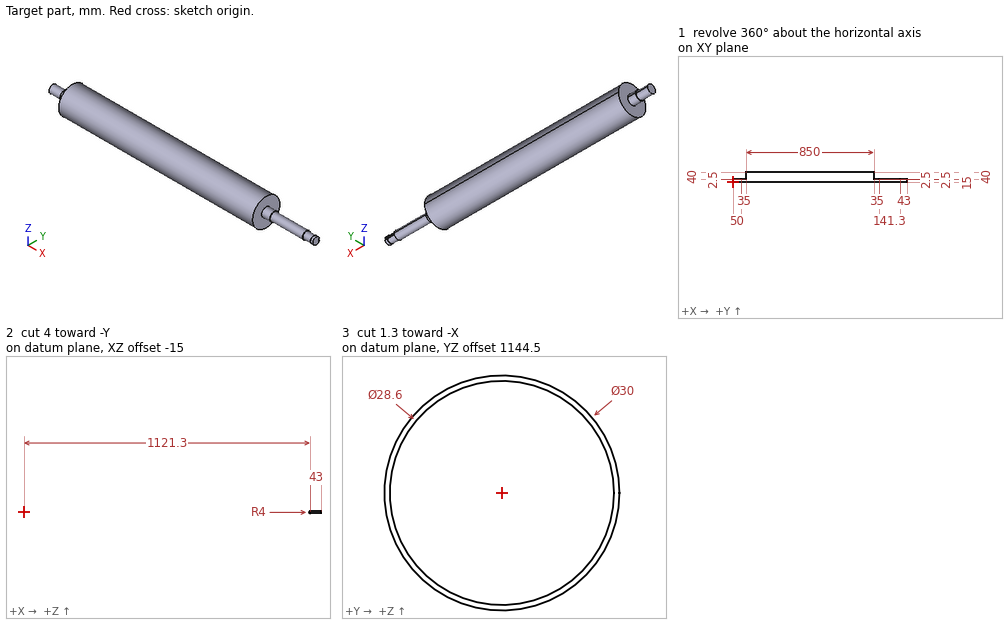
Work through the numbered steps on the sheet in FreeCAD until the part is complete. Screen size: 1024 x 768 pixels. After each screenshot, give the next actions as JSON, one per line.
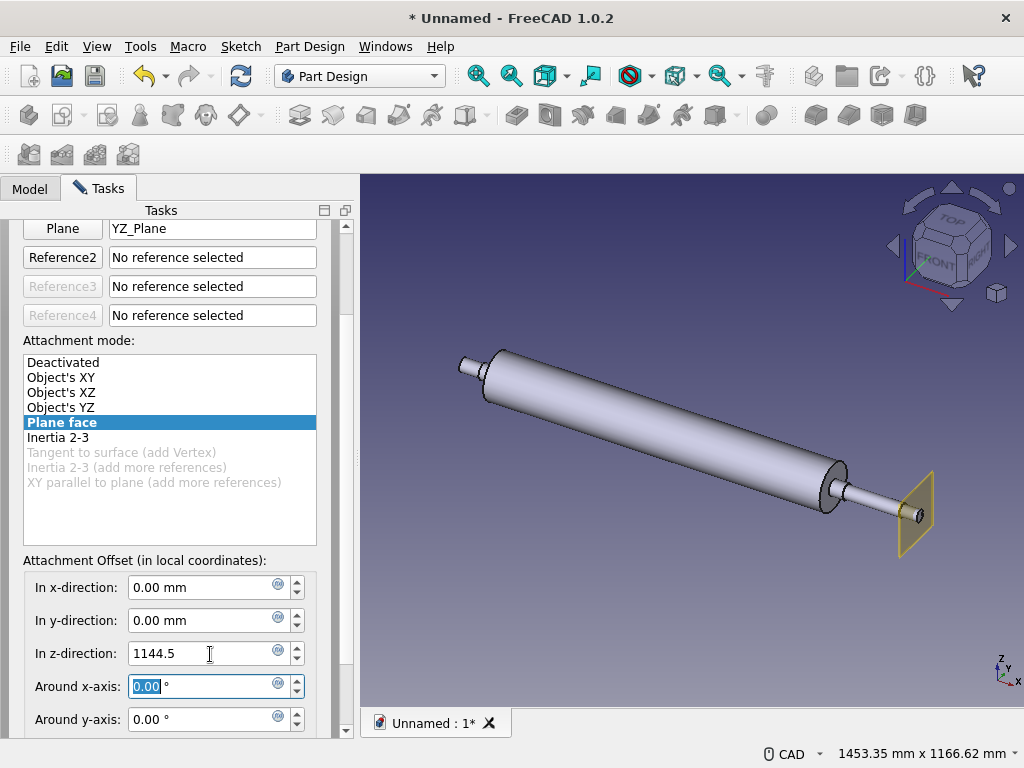
{"action": "scroll", "coordinate": [346, 479], "scroll_direction": "up", "scroll_amount": 3}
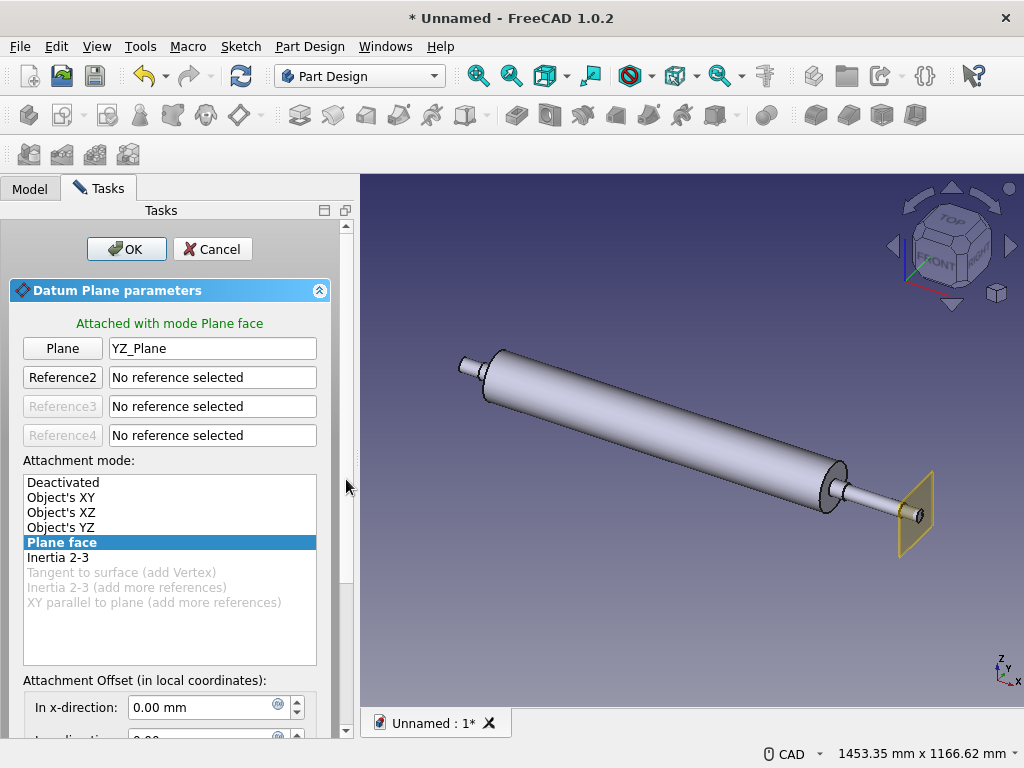
{"action": "left_click", "coordinate": [127, 249]}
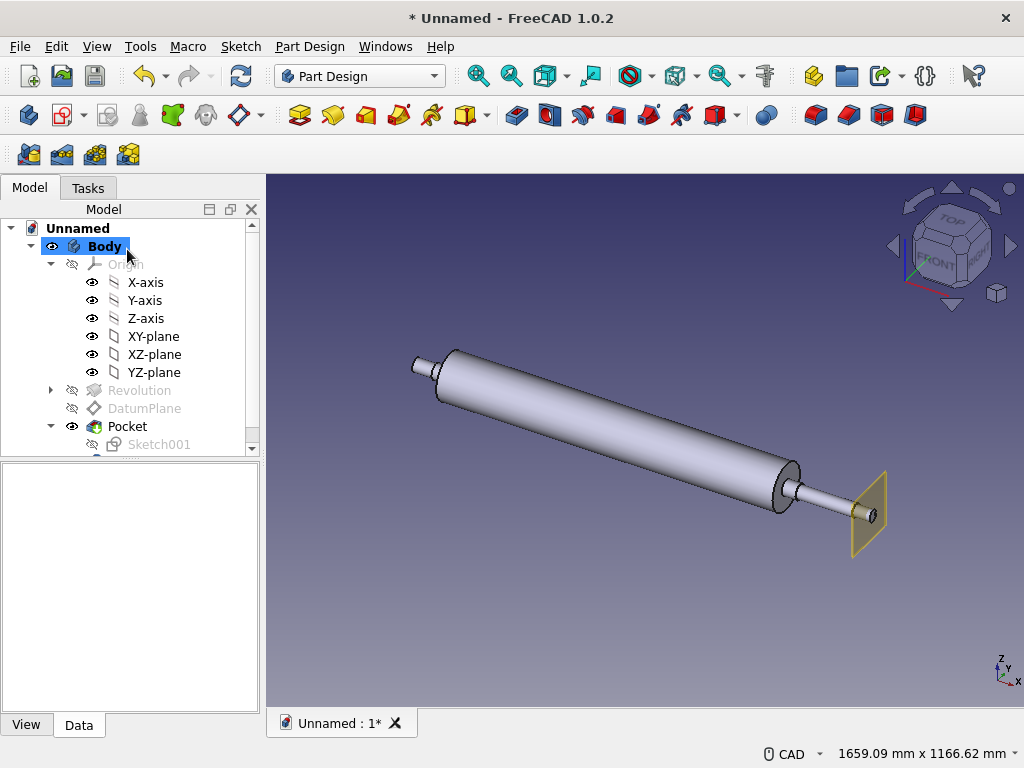
{"action": "scroll", "coordinate": [101, 332], "scroll_direction": "down", "scroll_amount": 3}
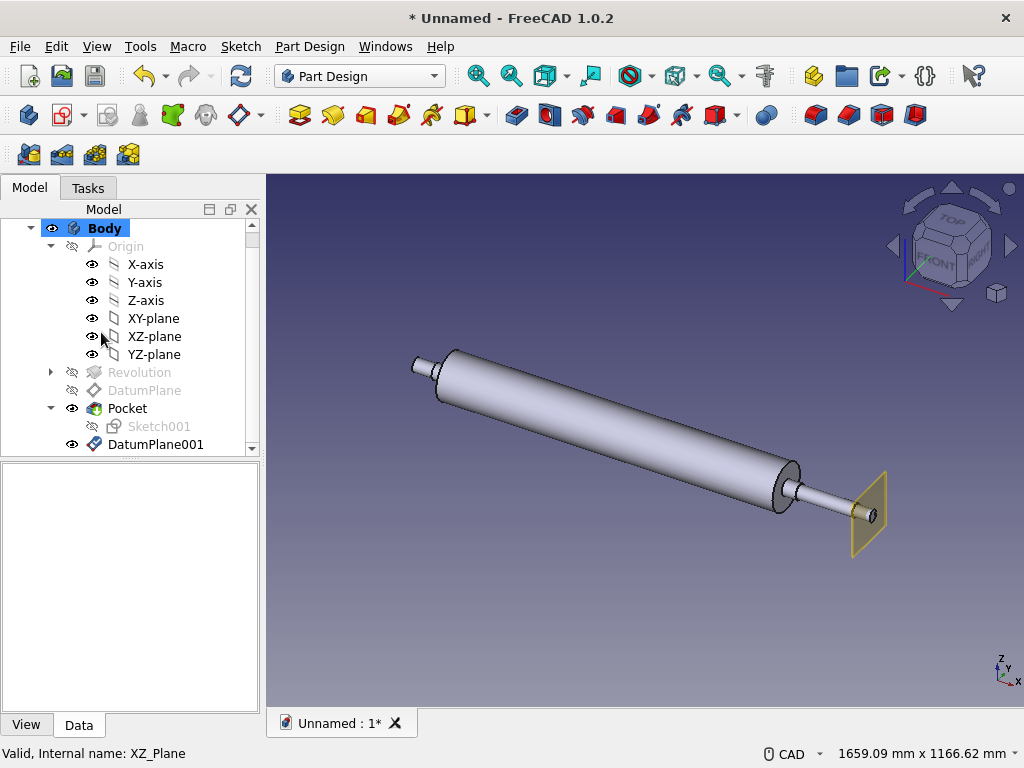
{"action": "left_click", "coordinate": [117, 444]}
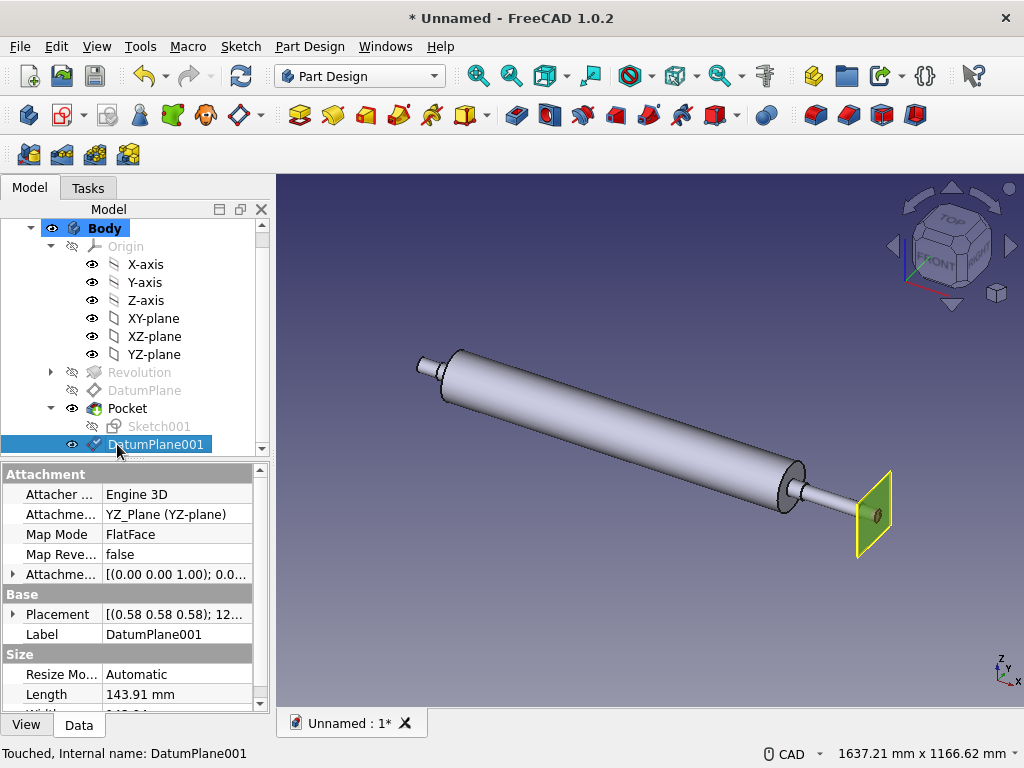
{"action": "left_click", "coordinate": [62, 116]}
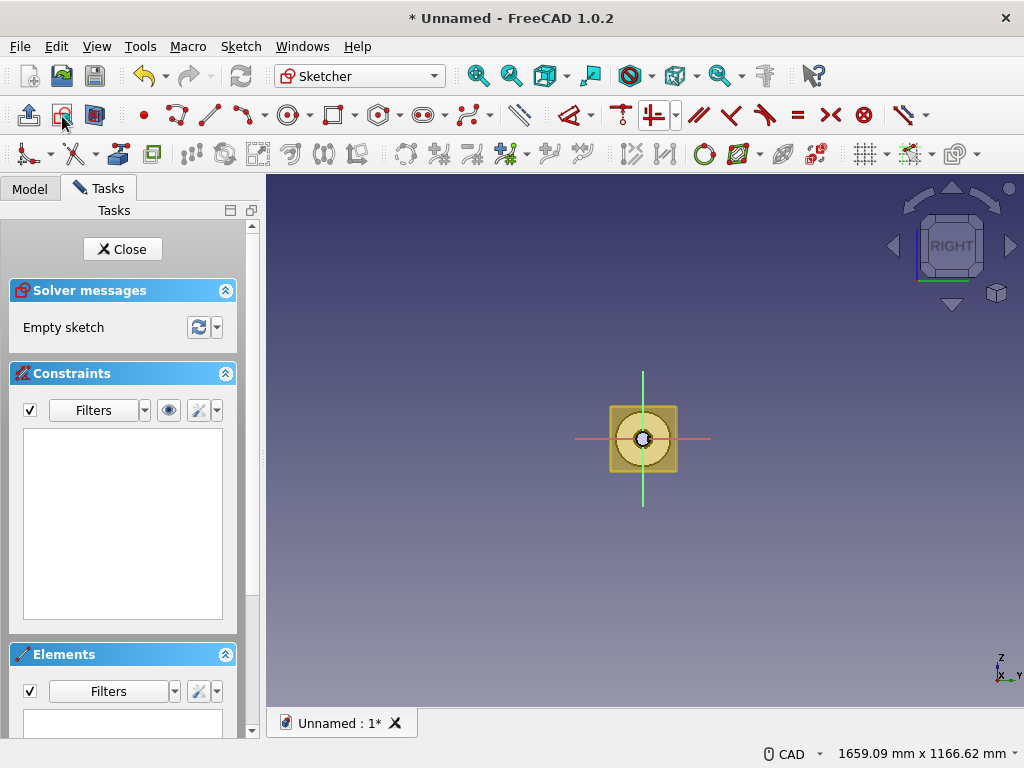
{"action": "key", "text": "q s"}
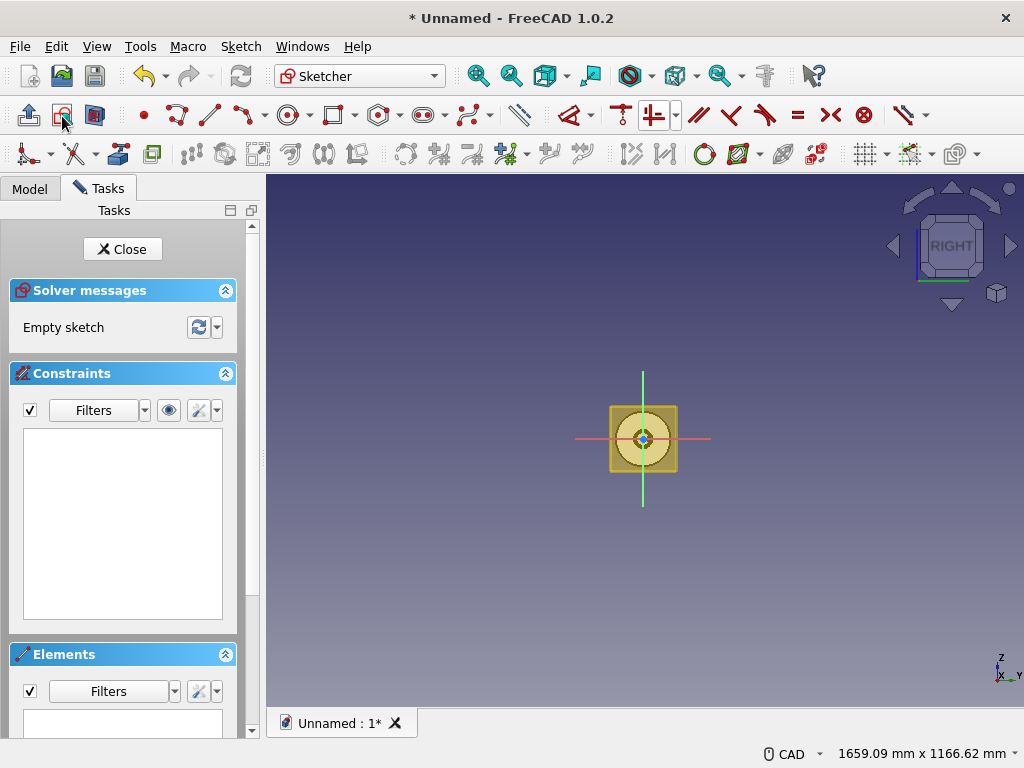
{"action": "scroll", "coordinate": [647, 439], "scroll_direction": "up", "scroll_amount": 15}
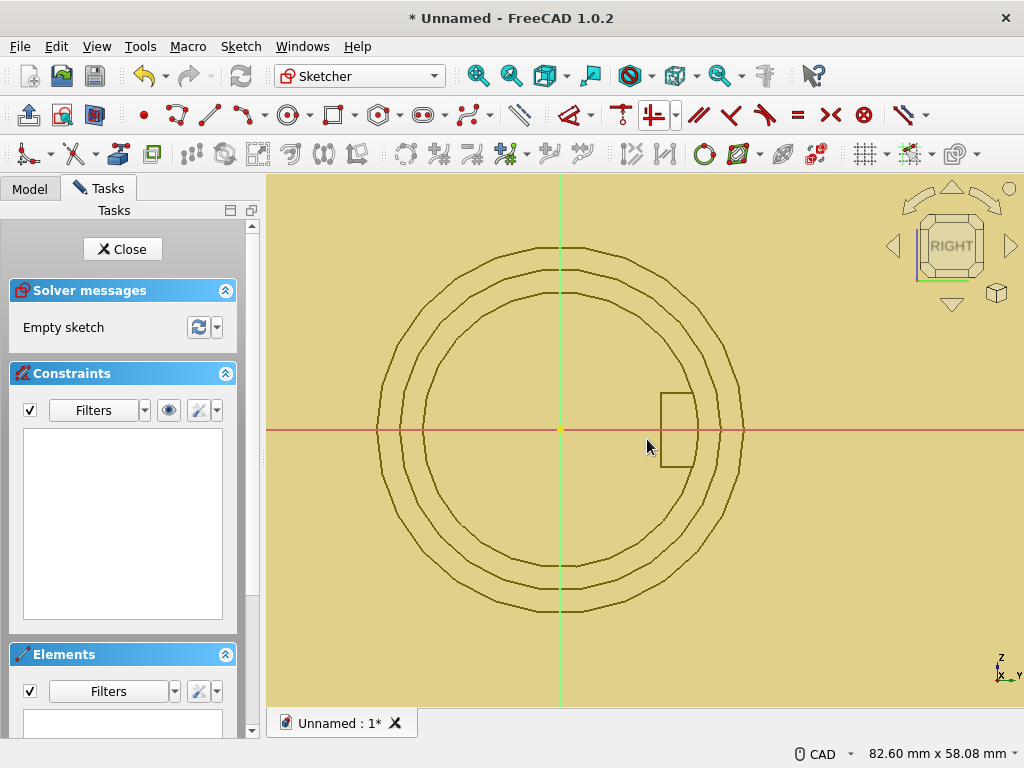
{"action": "left_click", "coordinate": [288, 116]}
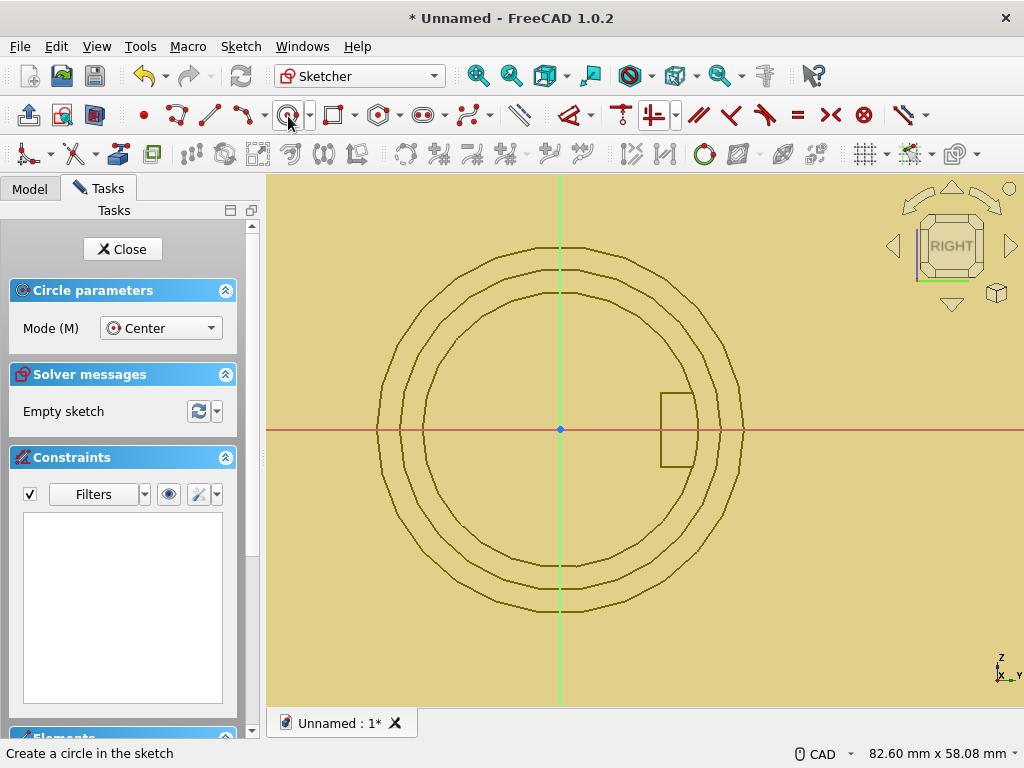
{"action": "left_click", "coordinate": [560, 430]}
{"action": "mouse_move", "coordinate": [658, 332]}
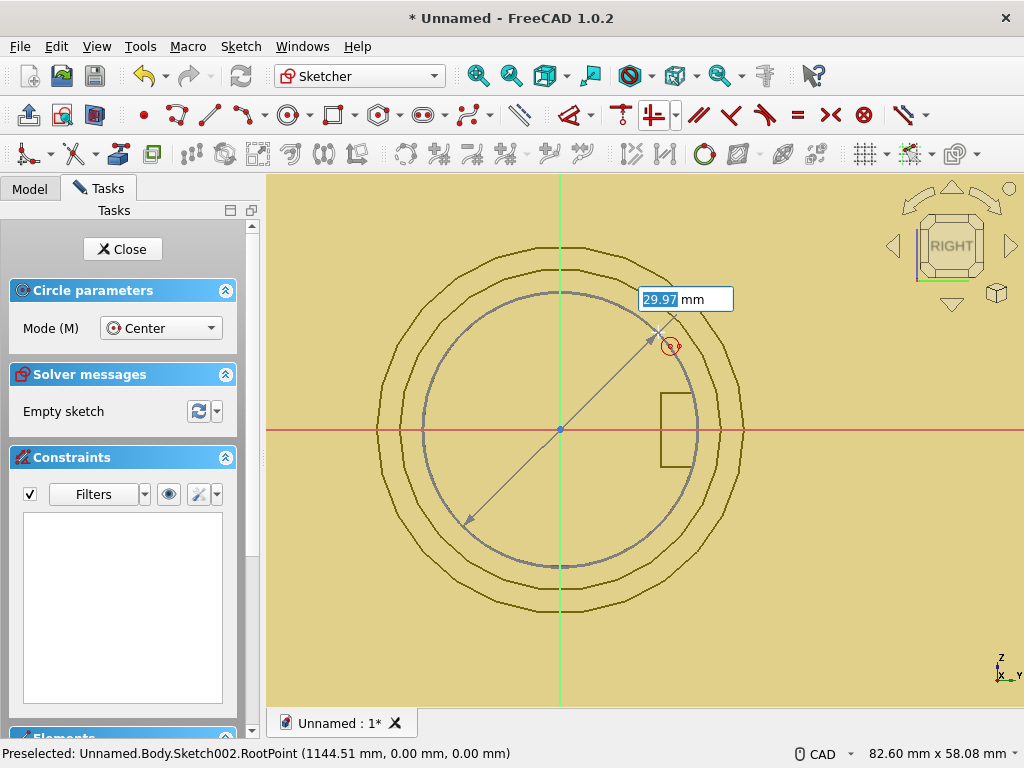
{"action": "type", "text": "30"}
{"action": "key", "text": "Return"}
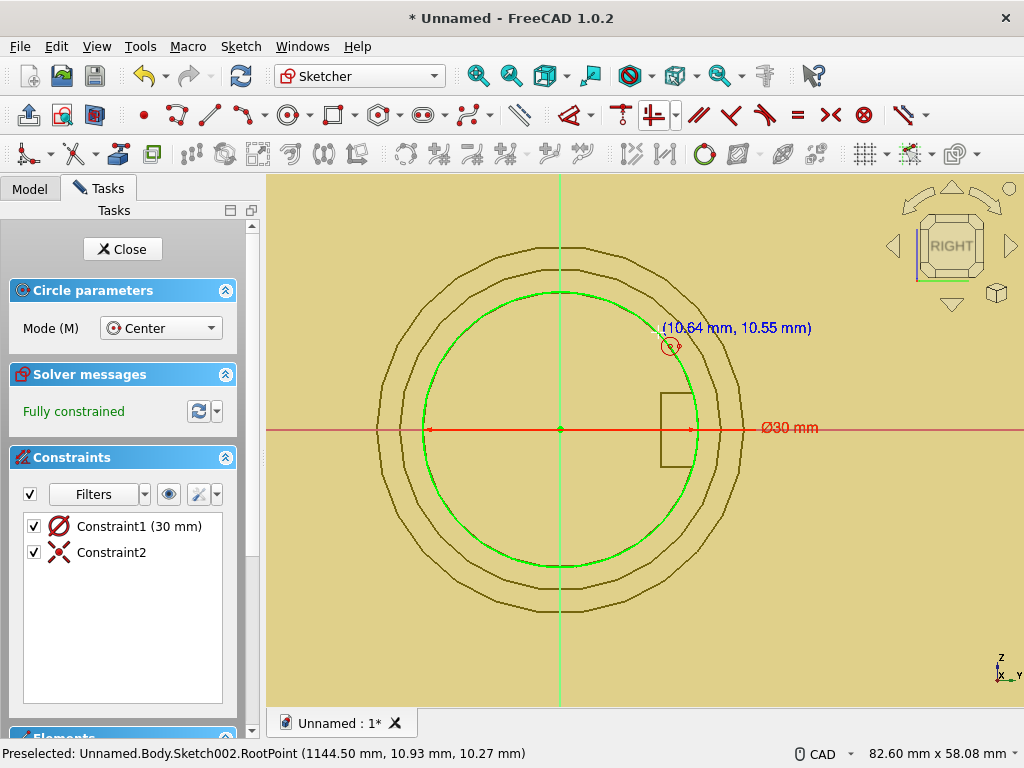
{"action": "left_click", "coordinate": [560, 430]}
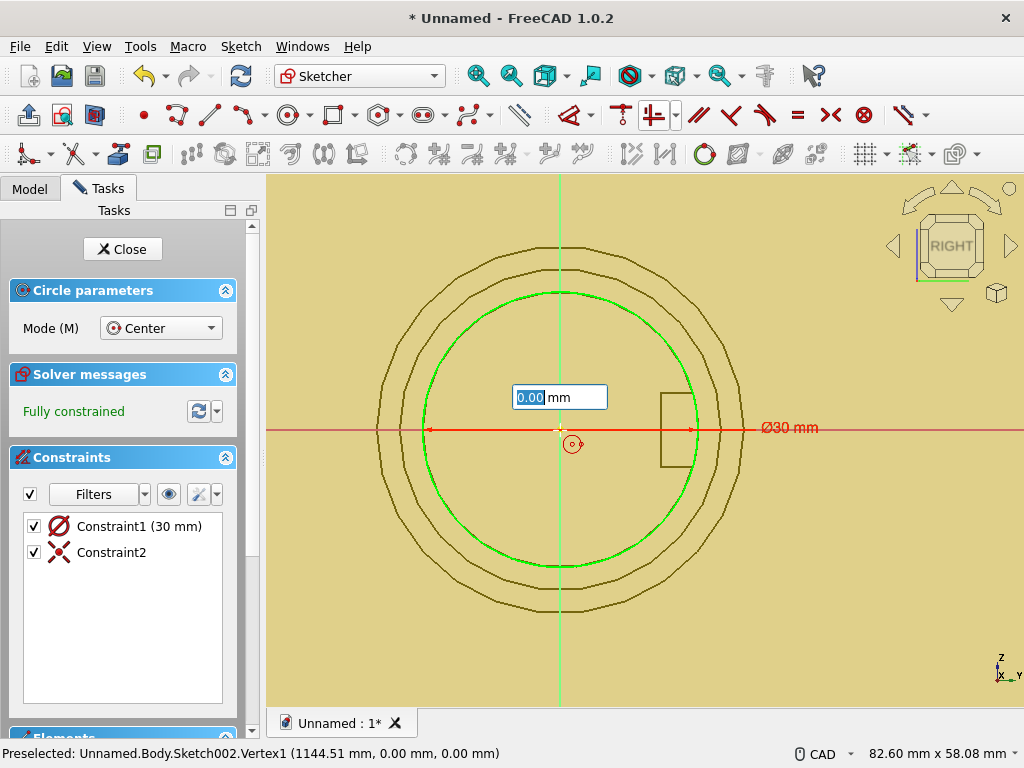
{"action": "scroll", "coordinate": [605, 306], "scroll_direction": "up", "scroll_amount": 5}
{"action": "mouse_move", "coordinate": [605, 307]}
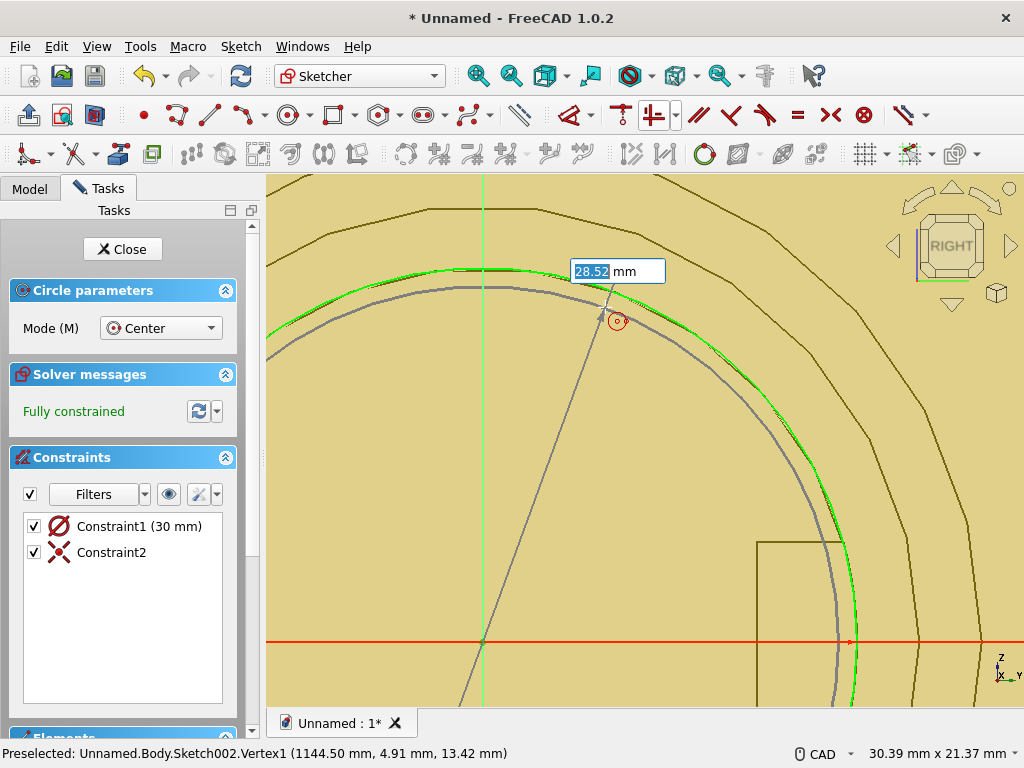
{"action": "type", "text": "28.6"}
{"action": "key", "text": "Return"}
{"action": "key", "text": "Escape"}